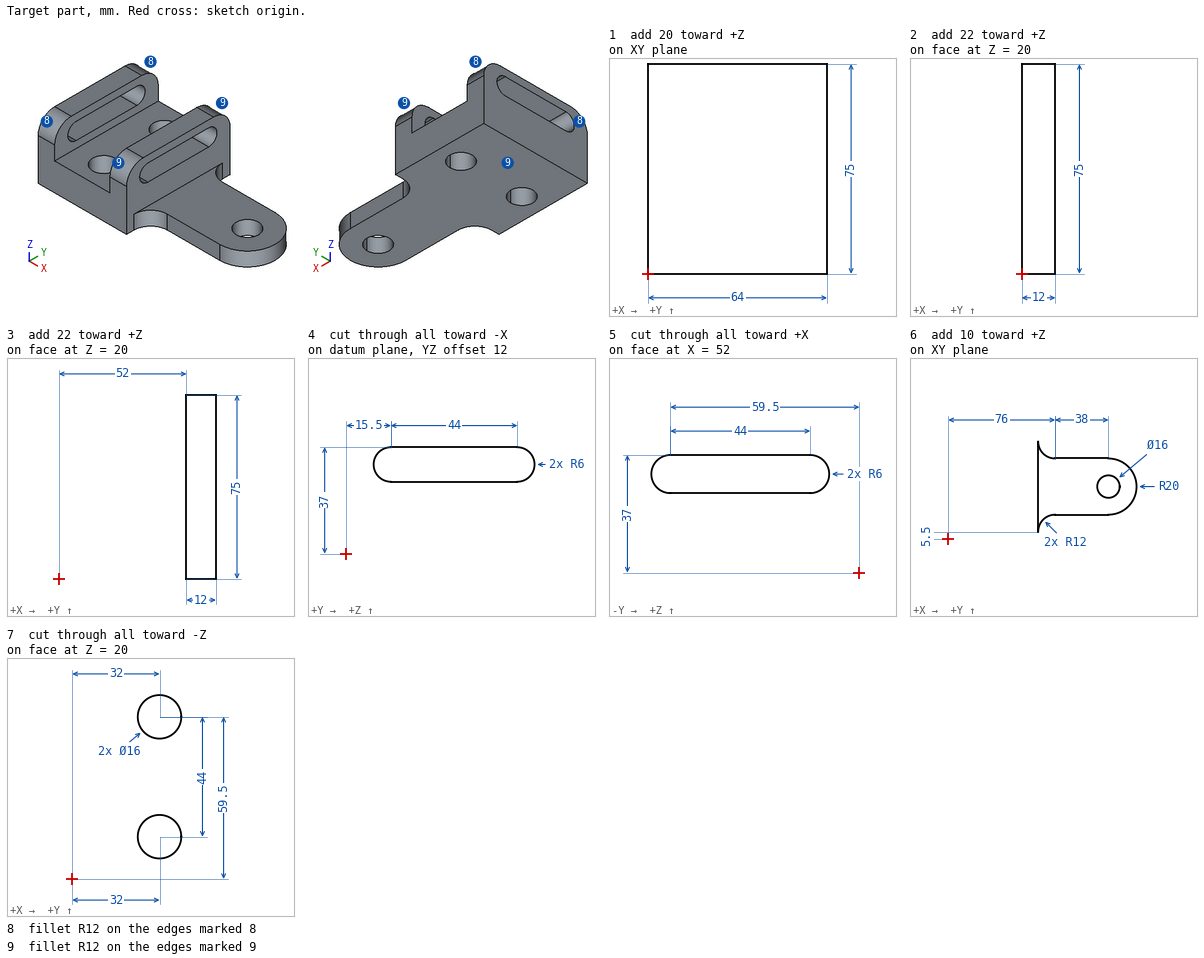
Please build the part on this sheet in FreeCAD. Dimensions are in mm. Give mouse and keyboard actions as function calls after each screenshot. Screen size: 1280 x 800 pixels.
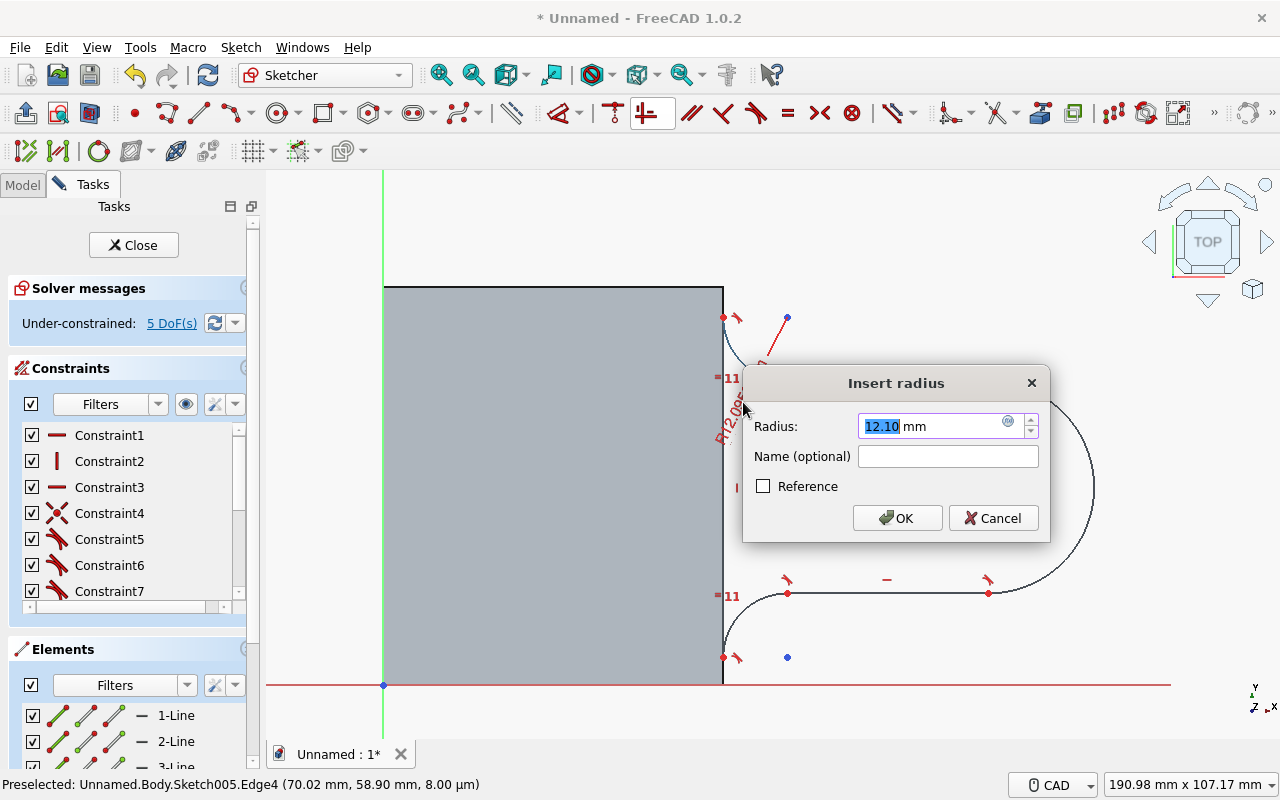
text(12)
key(Return)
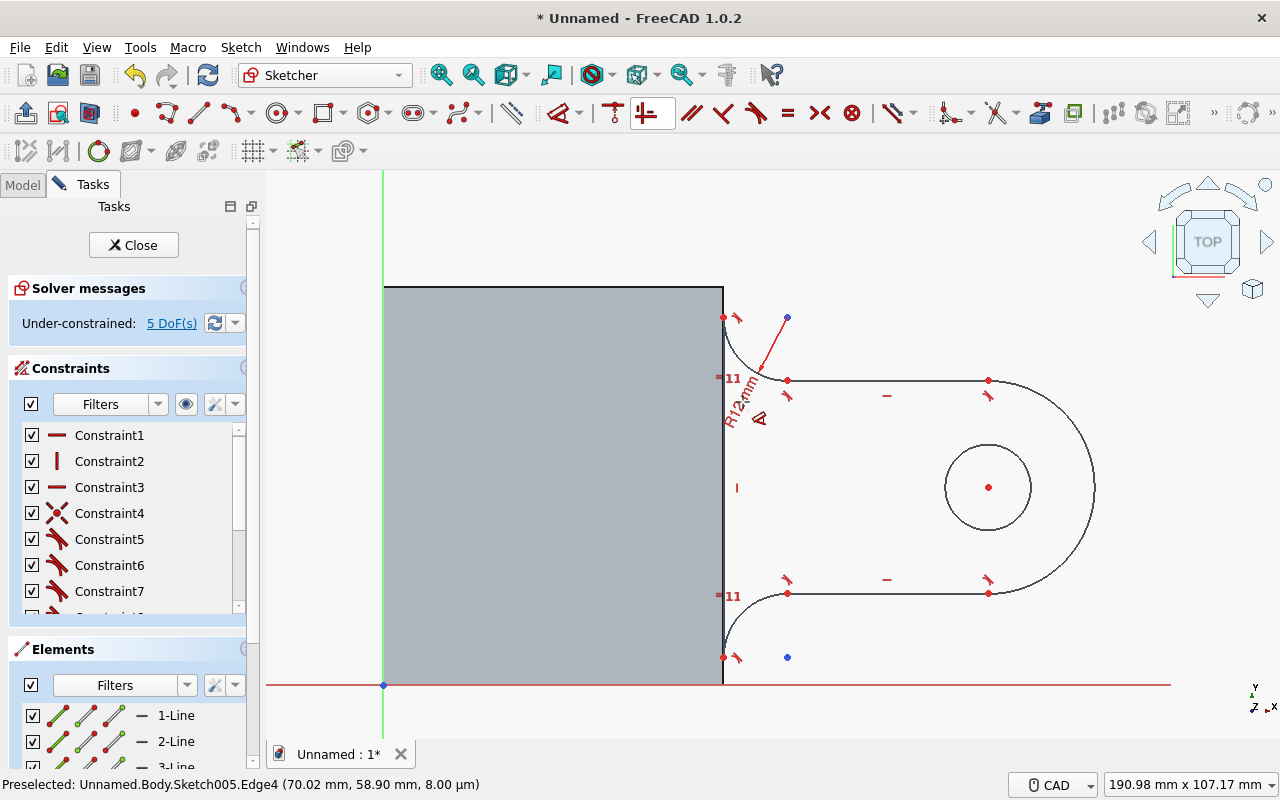
click(1074, 550)
click(1100, 569)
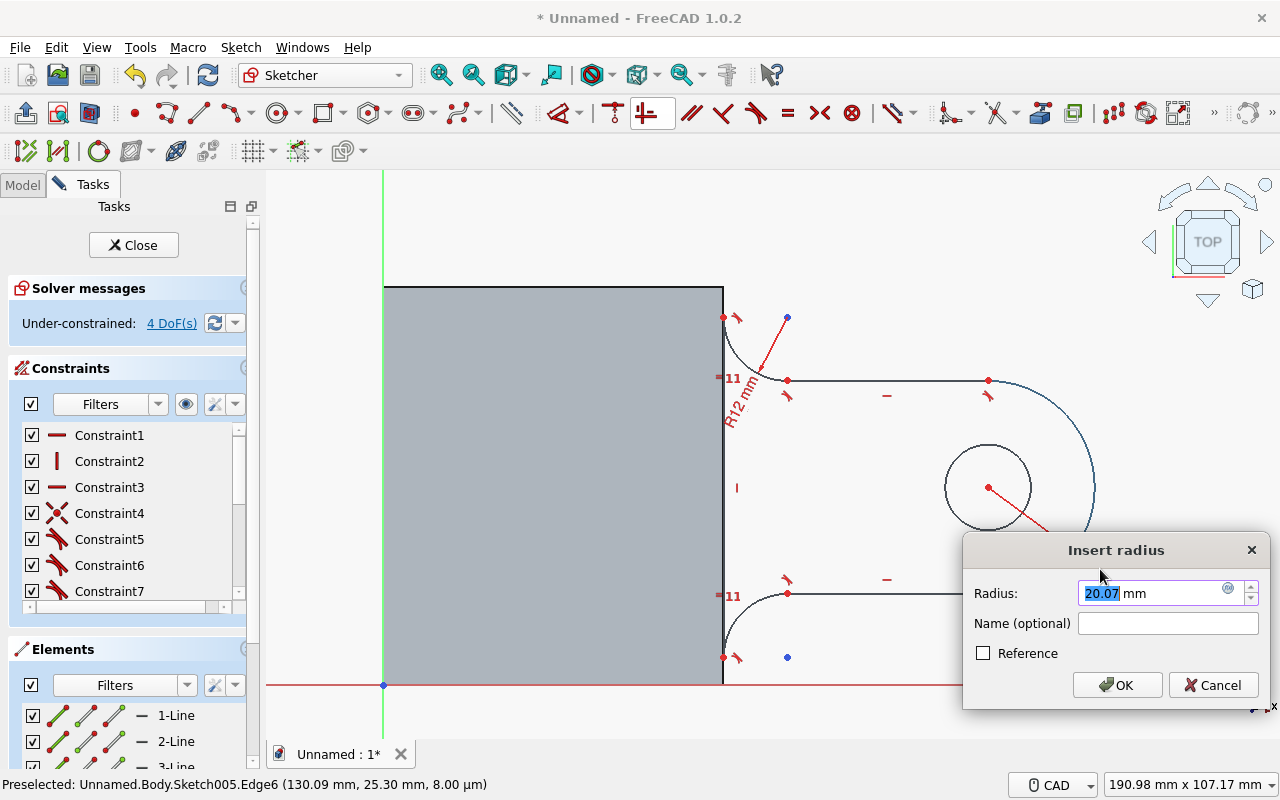
text(20)
key(Return)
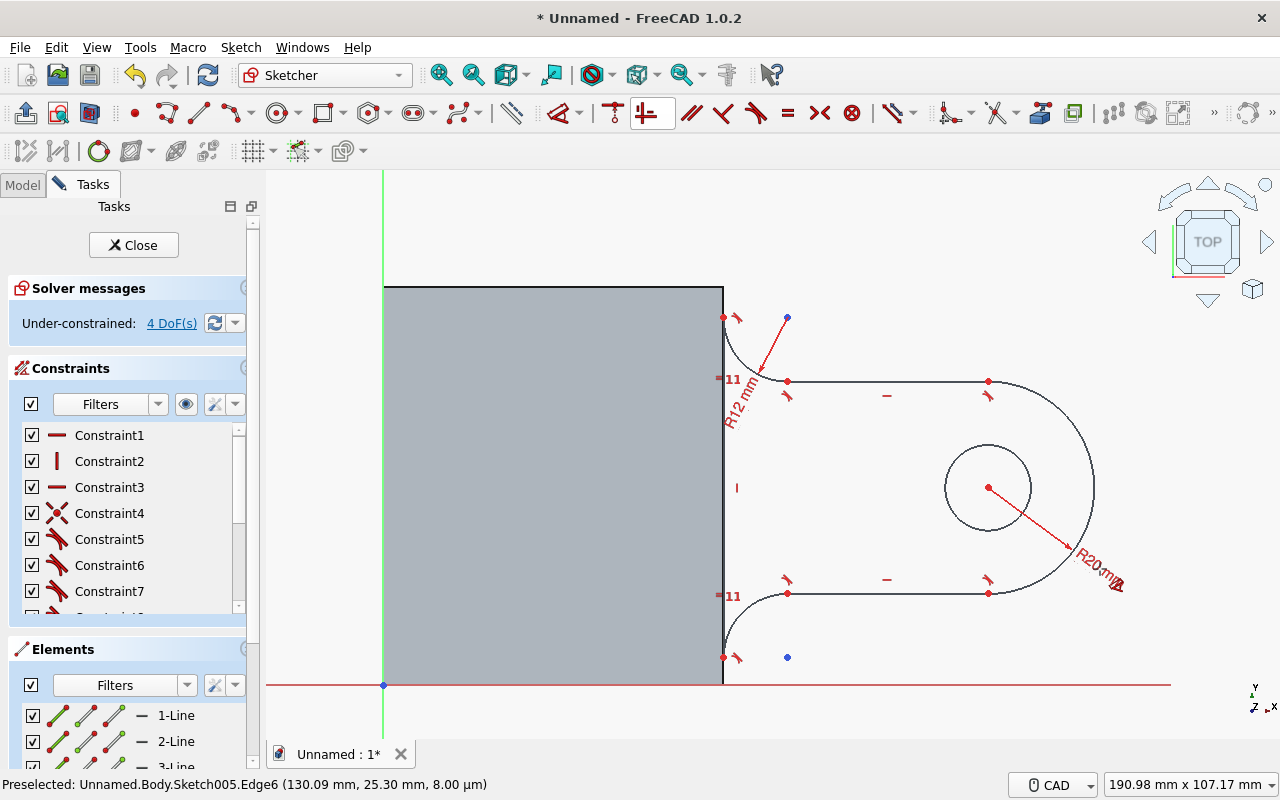
click(1018, 457)
click(1040, 434)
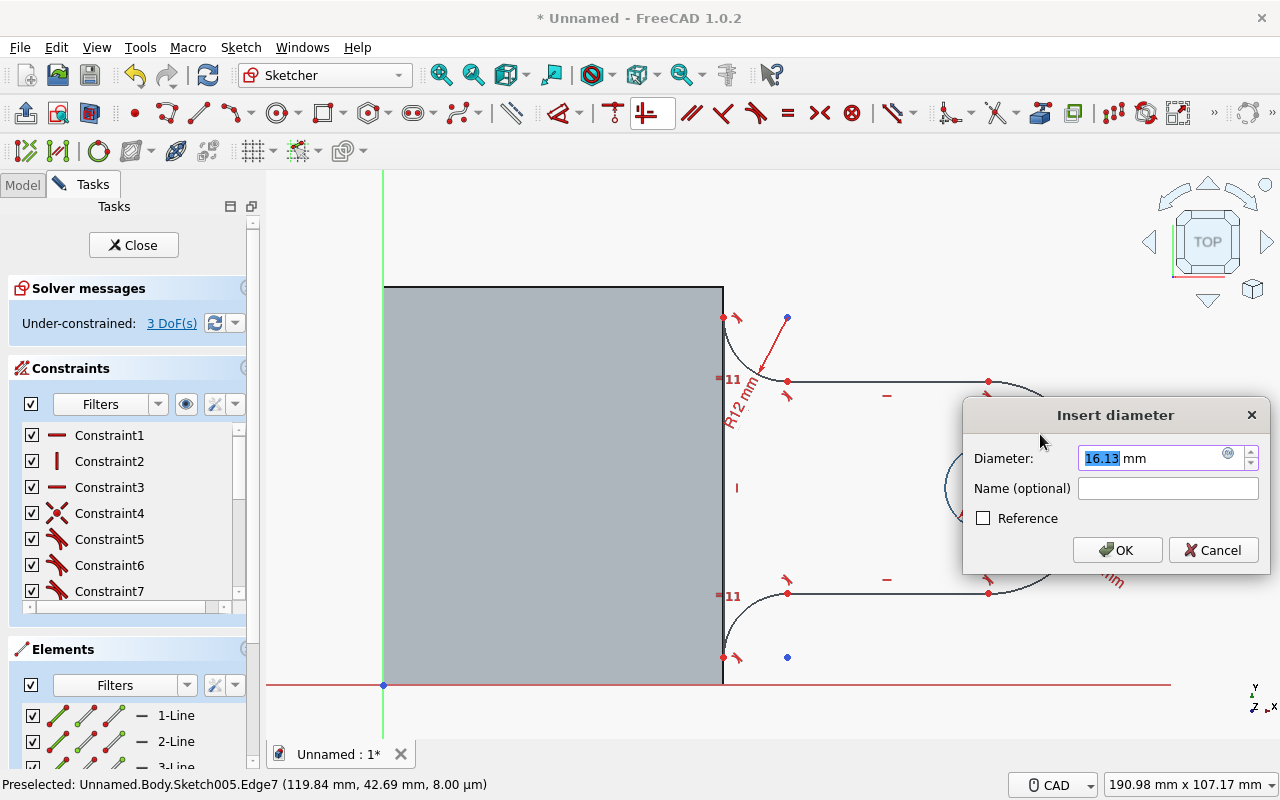
text(16)
key(Return)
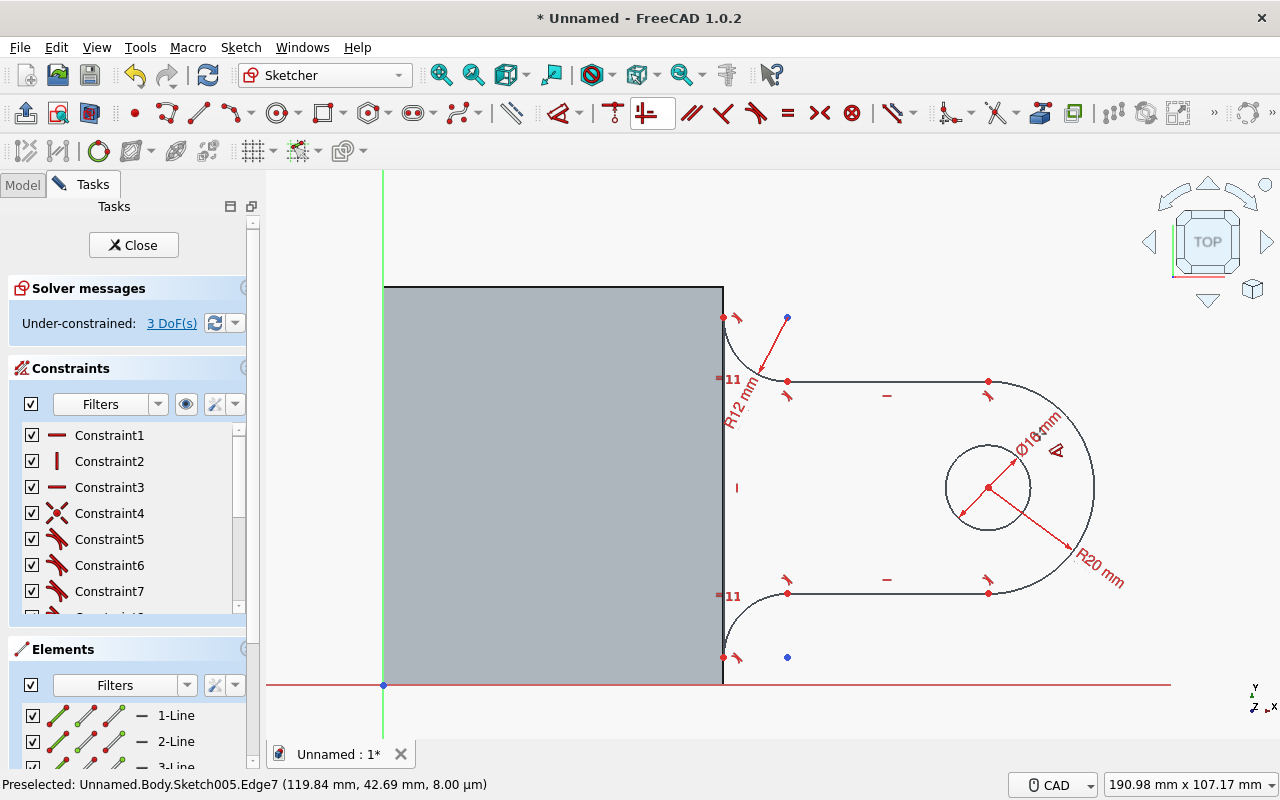
click(928, 382)
click(888, 348)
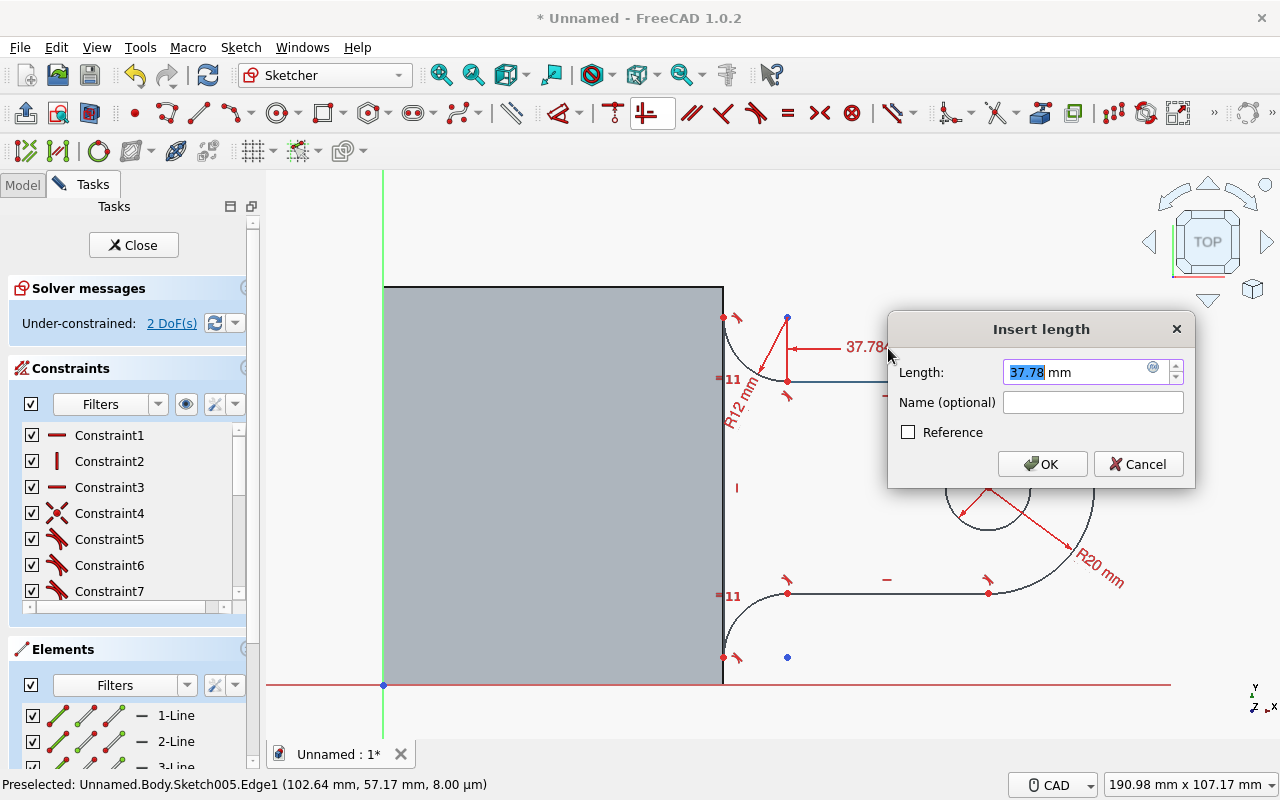
text(38)
key(Return)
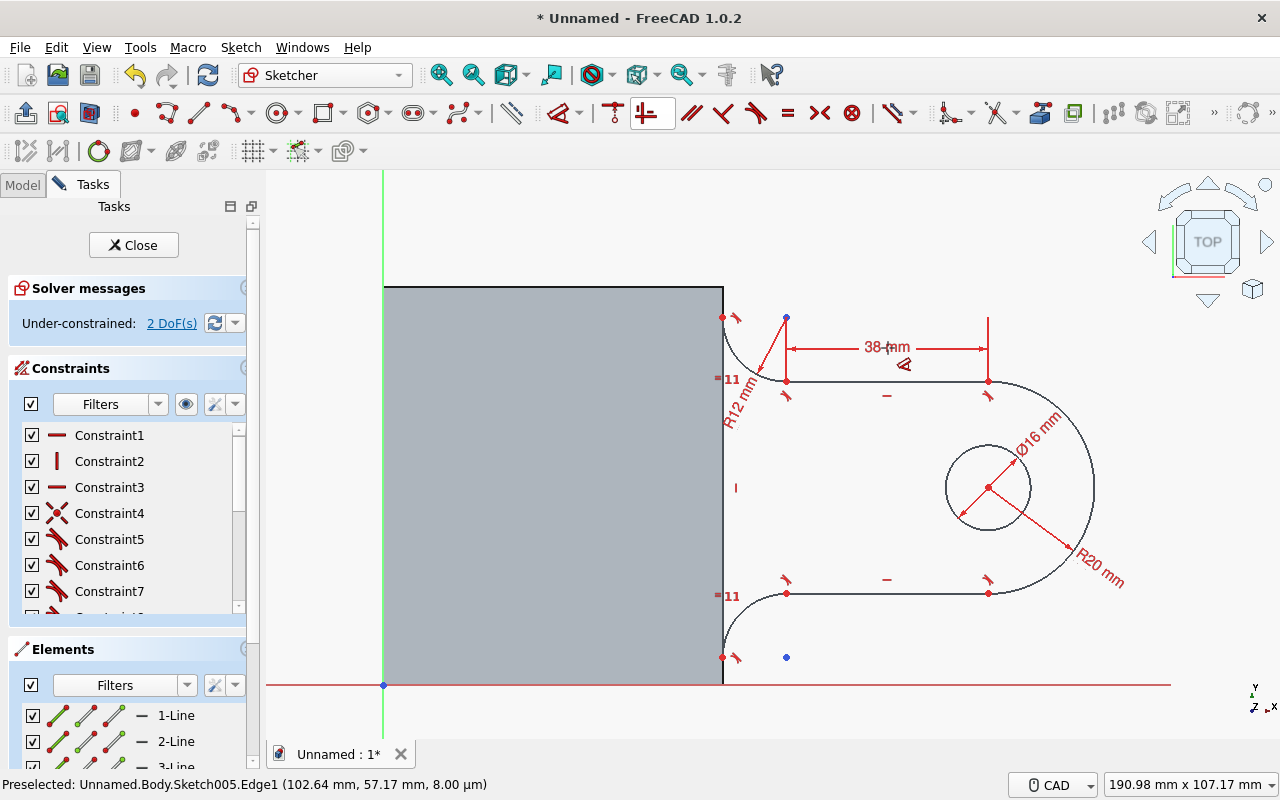
click(786, 382)
click(585, 348)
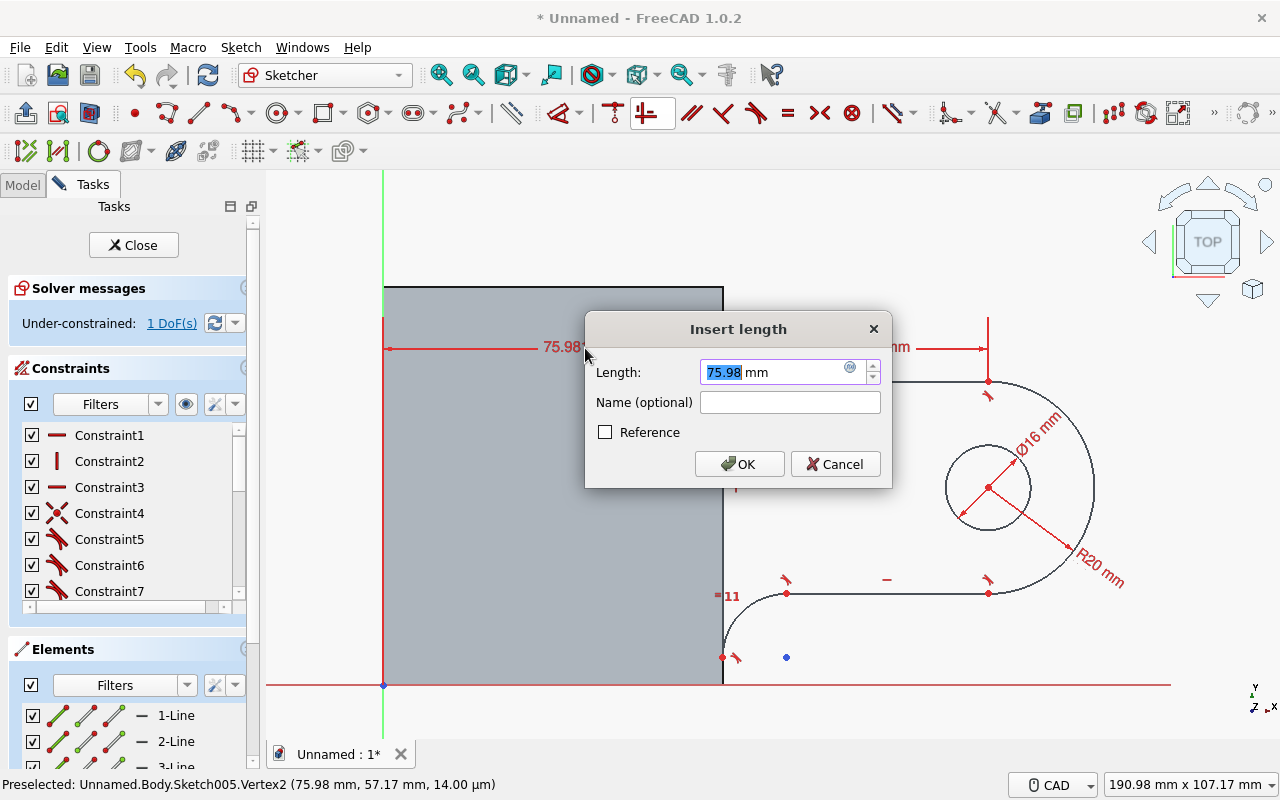
text(76)
key(Return)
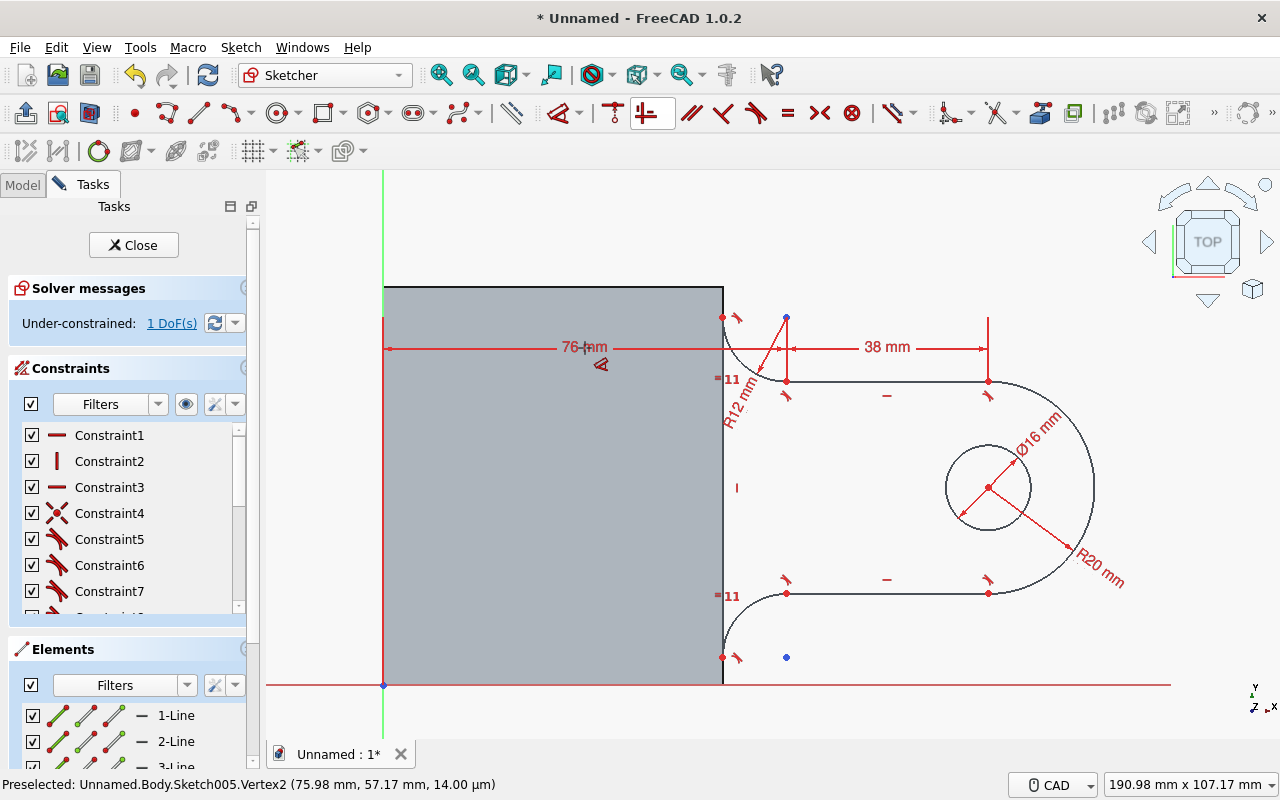
scroll(723, 658, up, 2)